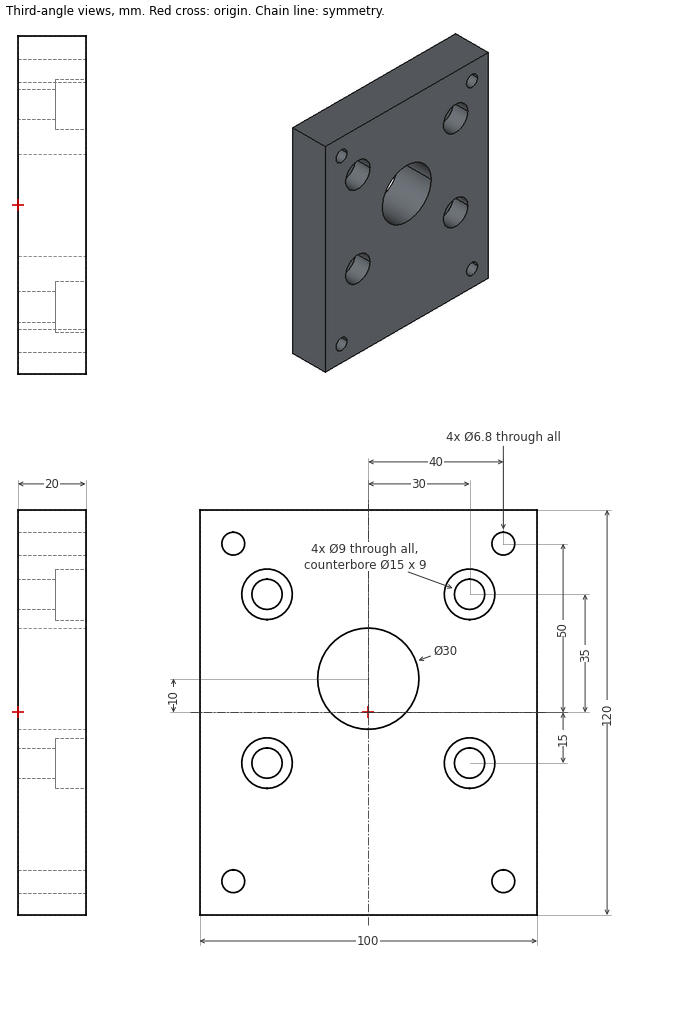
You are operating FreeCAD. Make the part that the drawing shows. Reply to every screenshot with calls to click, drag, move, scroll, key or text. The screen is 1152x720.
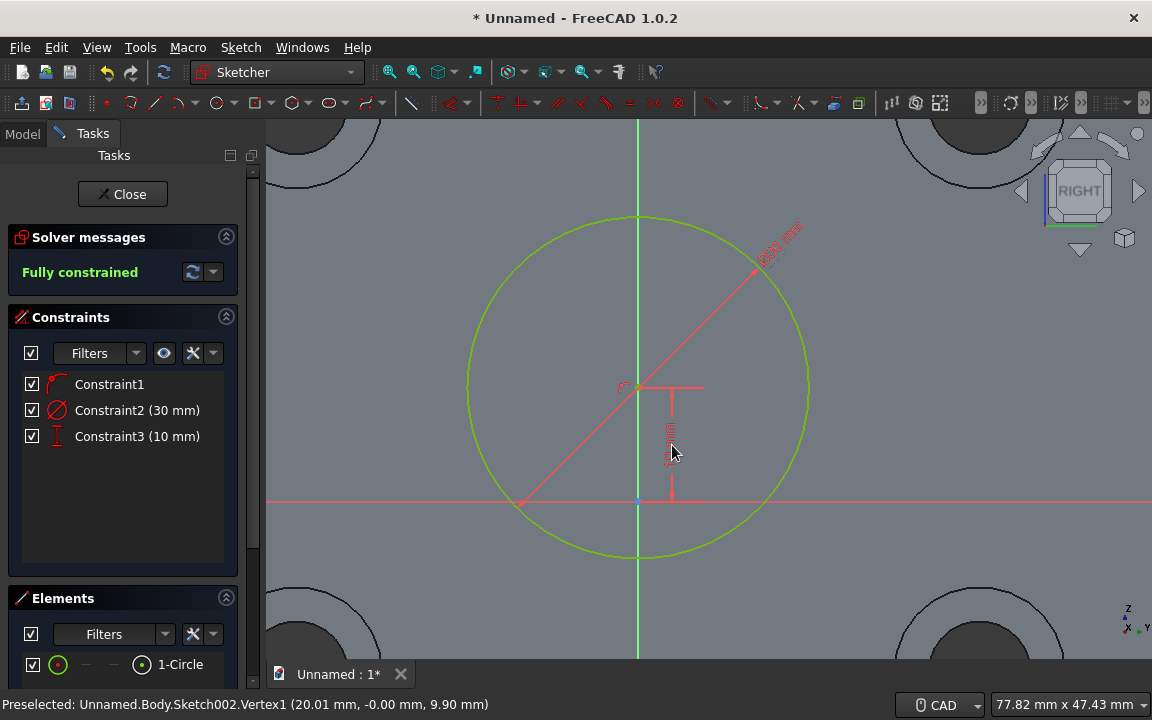
click(123, 194)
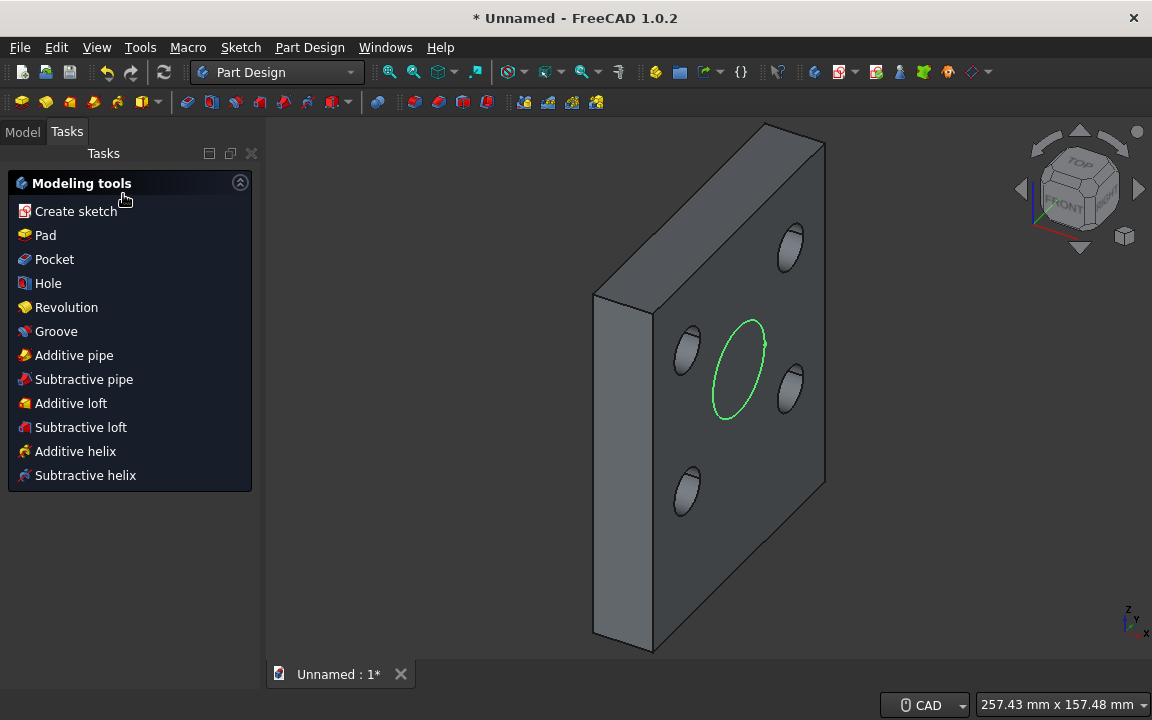
click(188, 102)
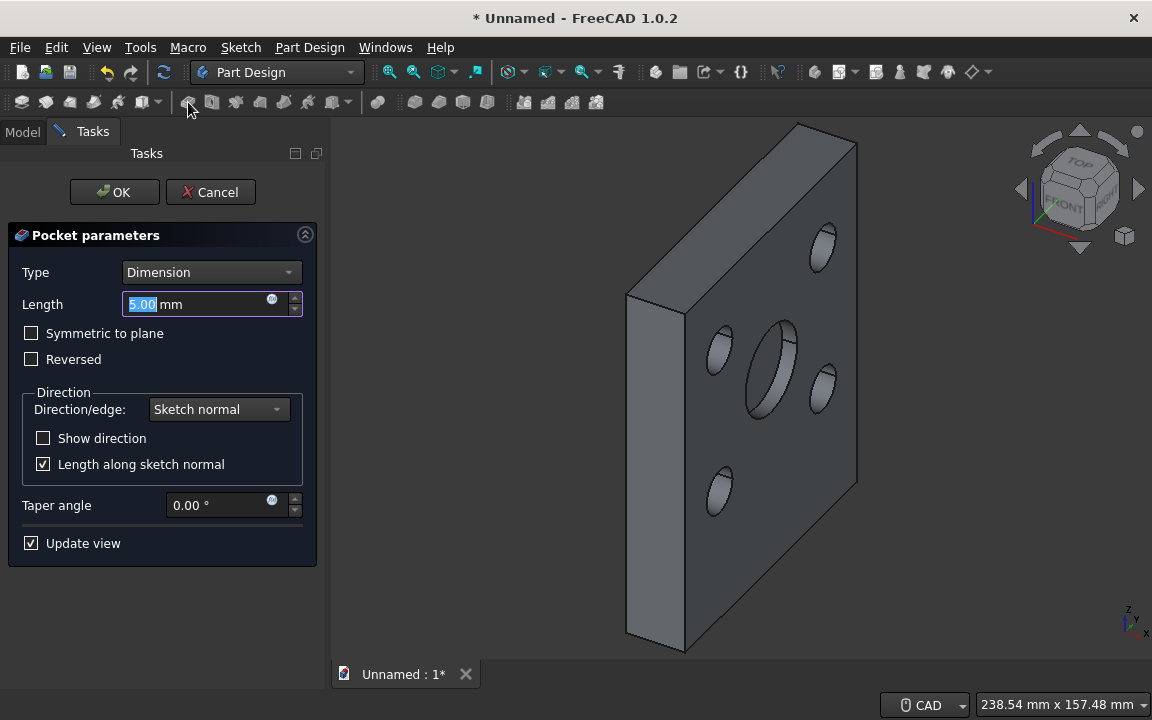
click(212, 272)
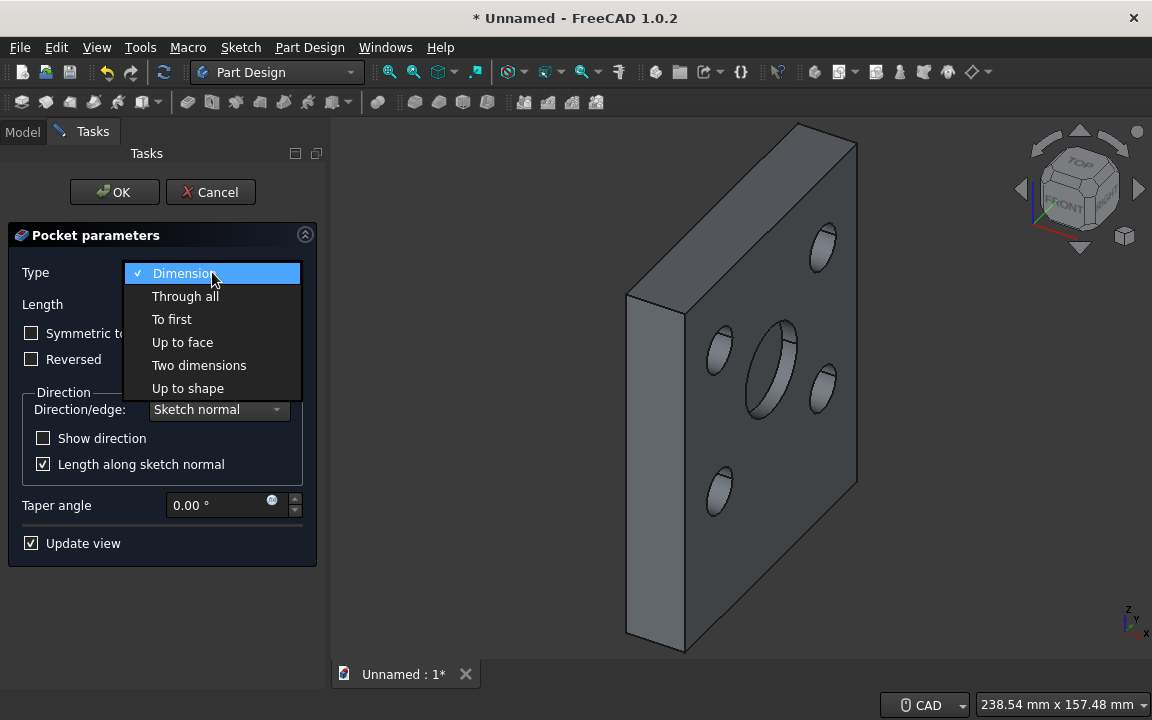
click(212, 296)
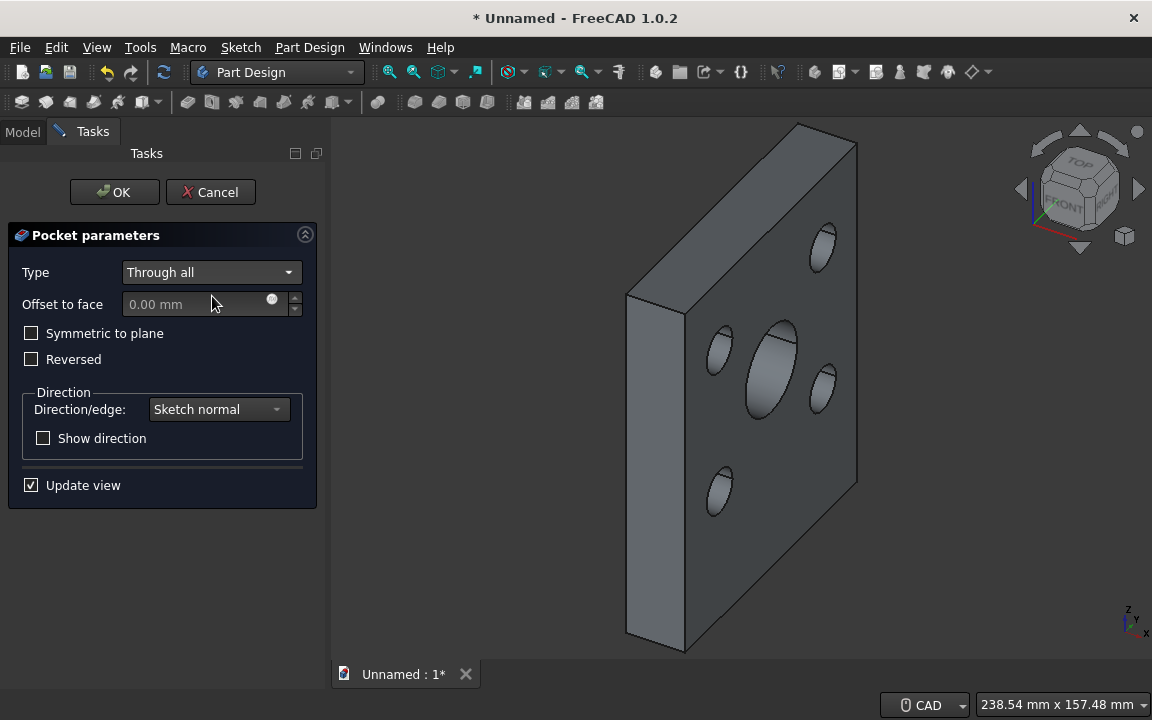
click(115, 192)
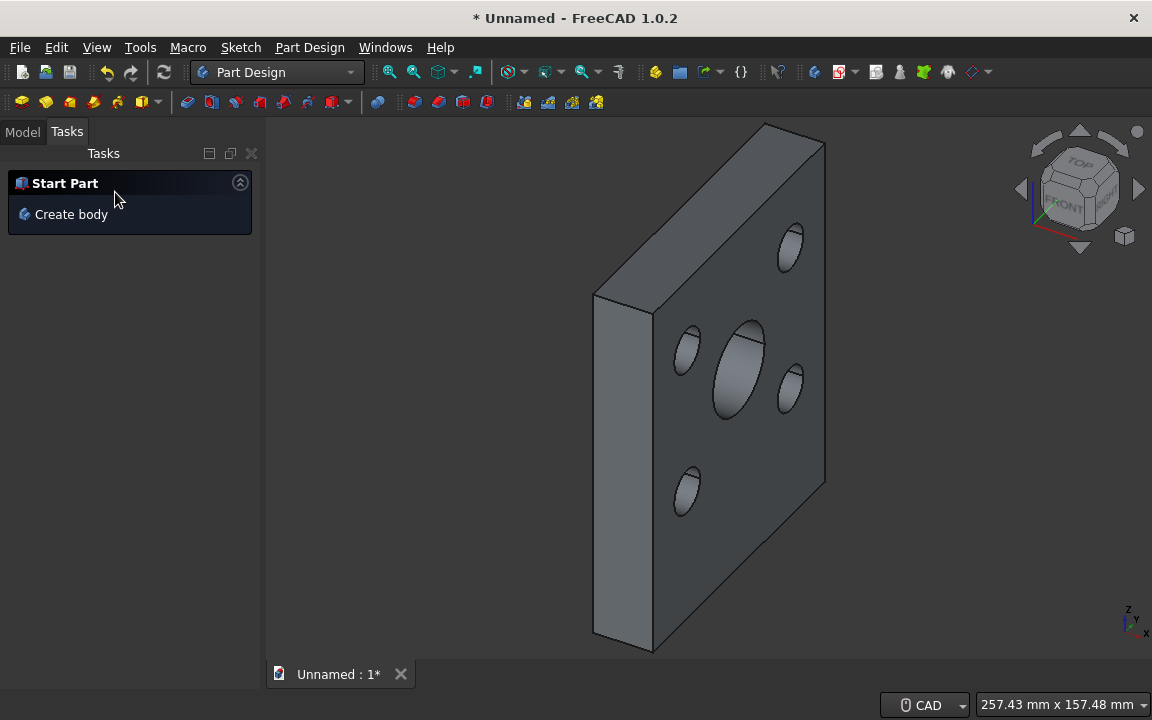
click(739, 494)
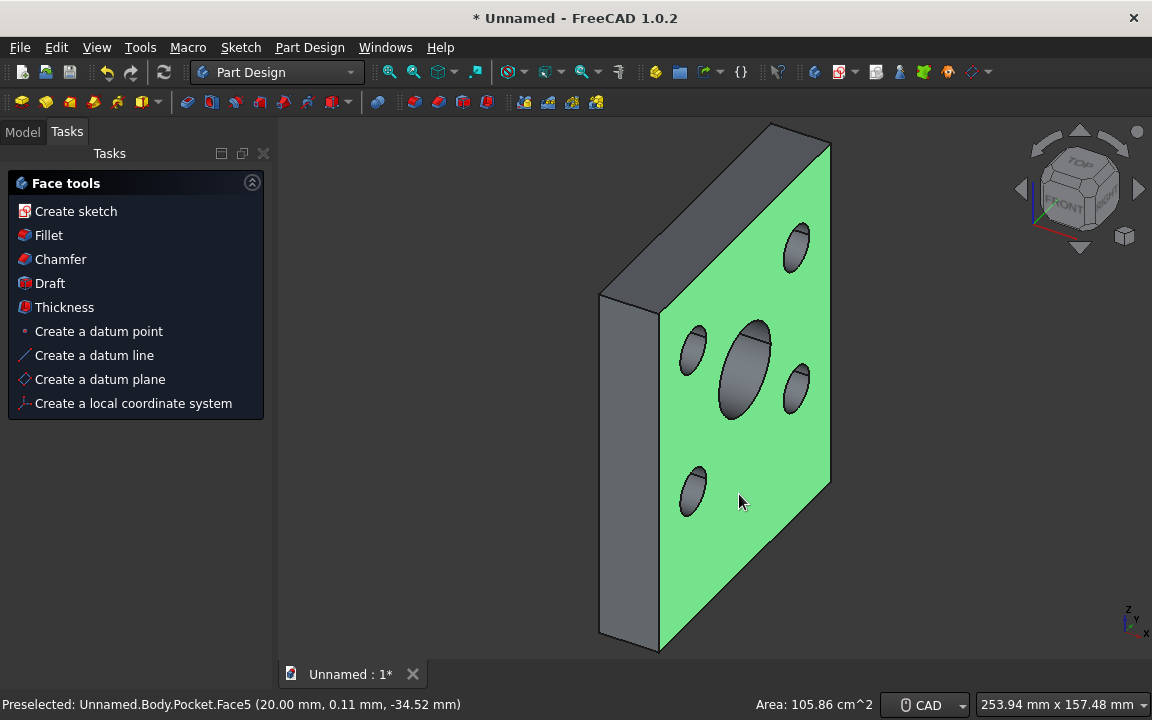
click(840, 72)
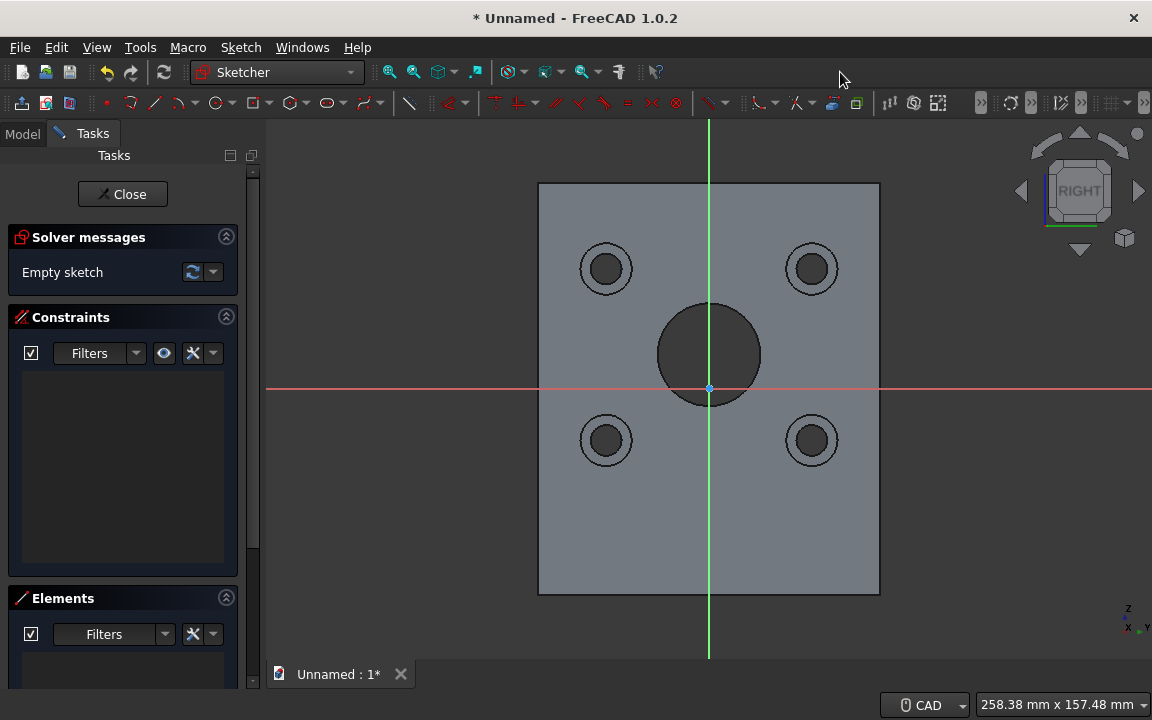
click(216, 104)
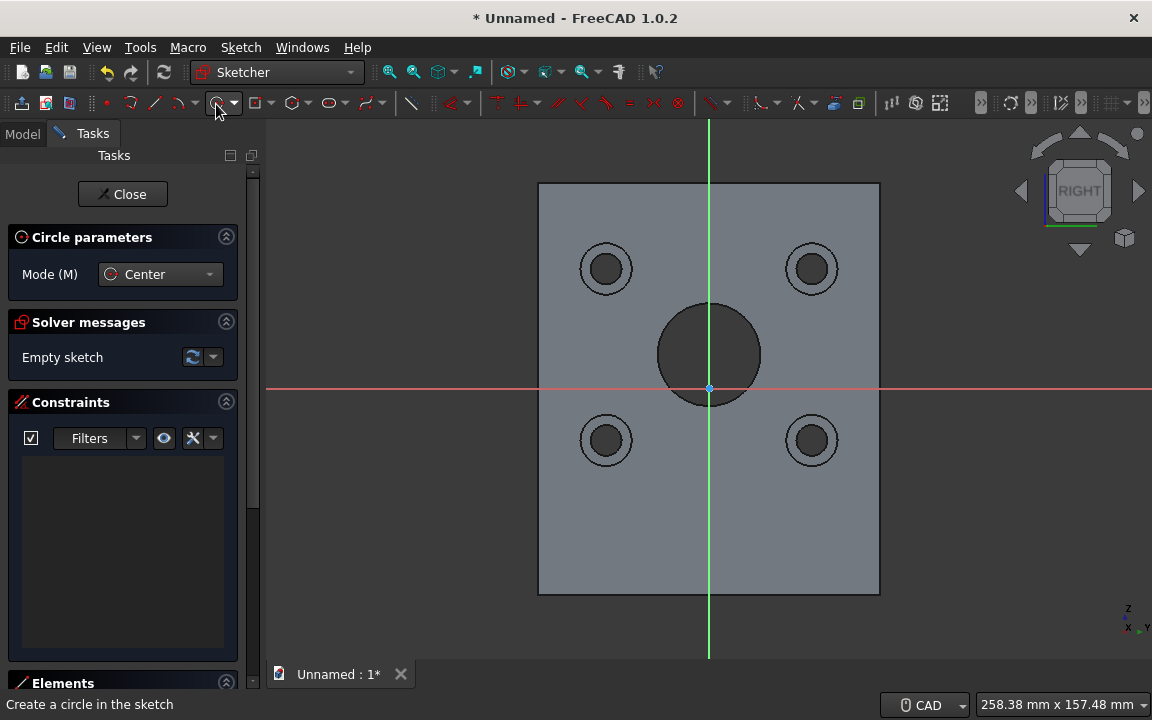
scroll(846, 218, up, 4)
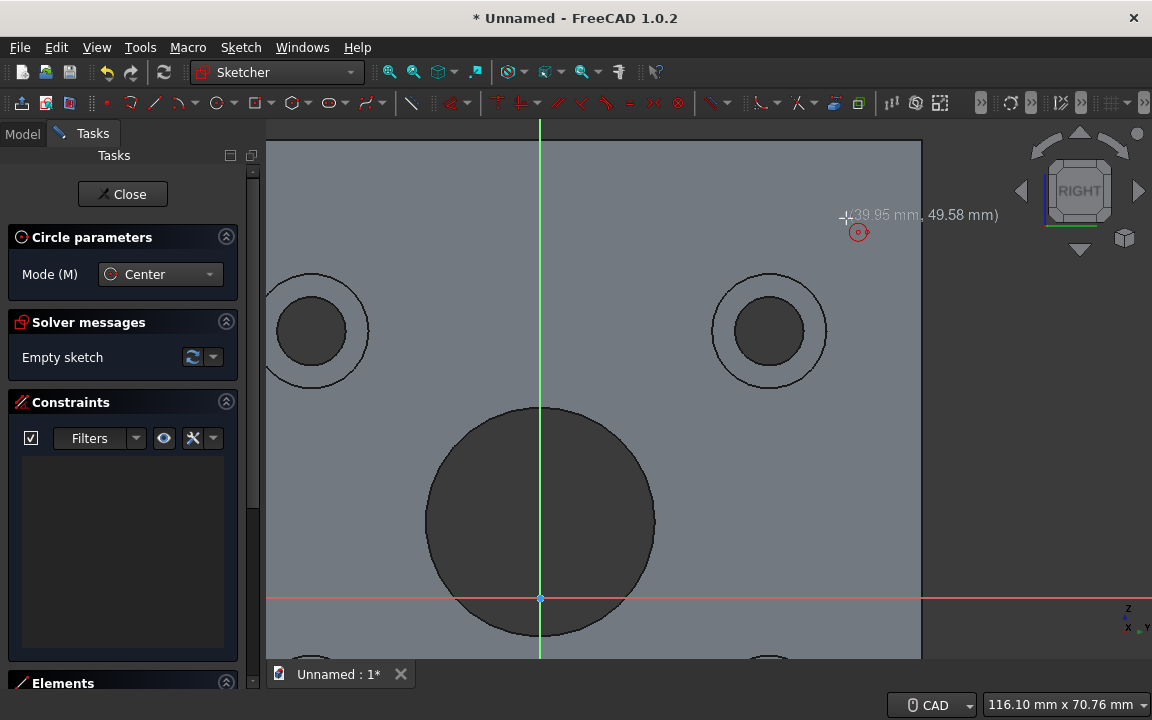
click(846, 217)
click(864, 198)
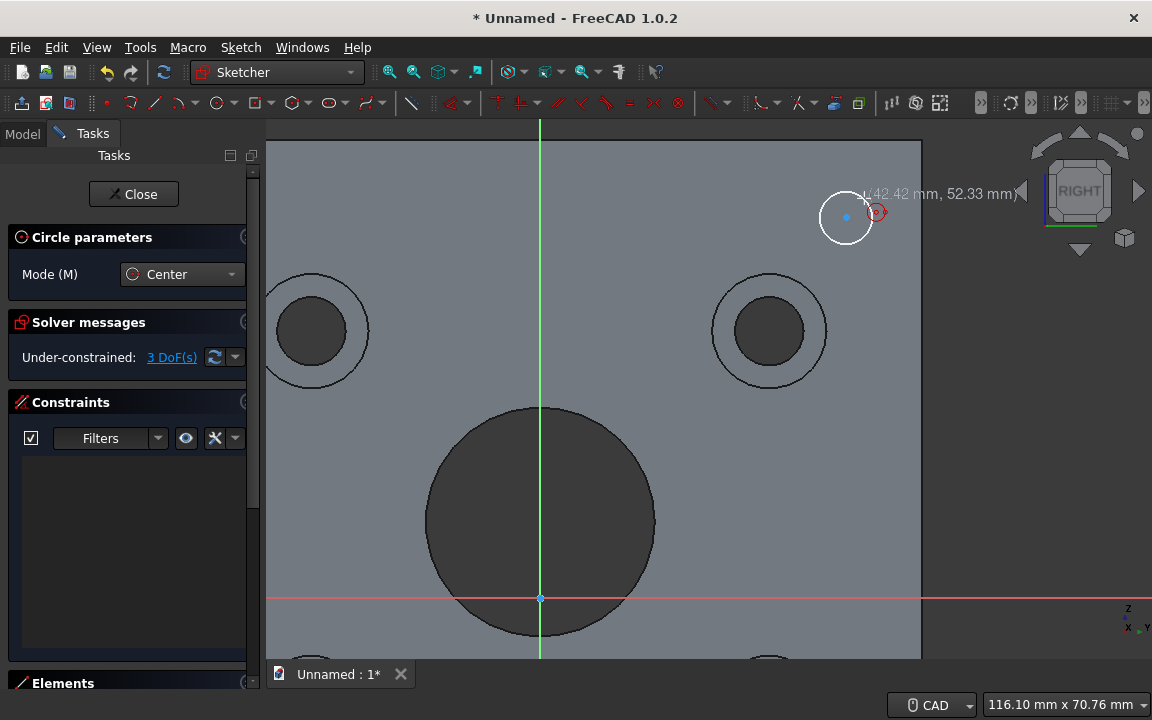
scroll(722, 218, down, 4)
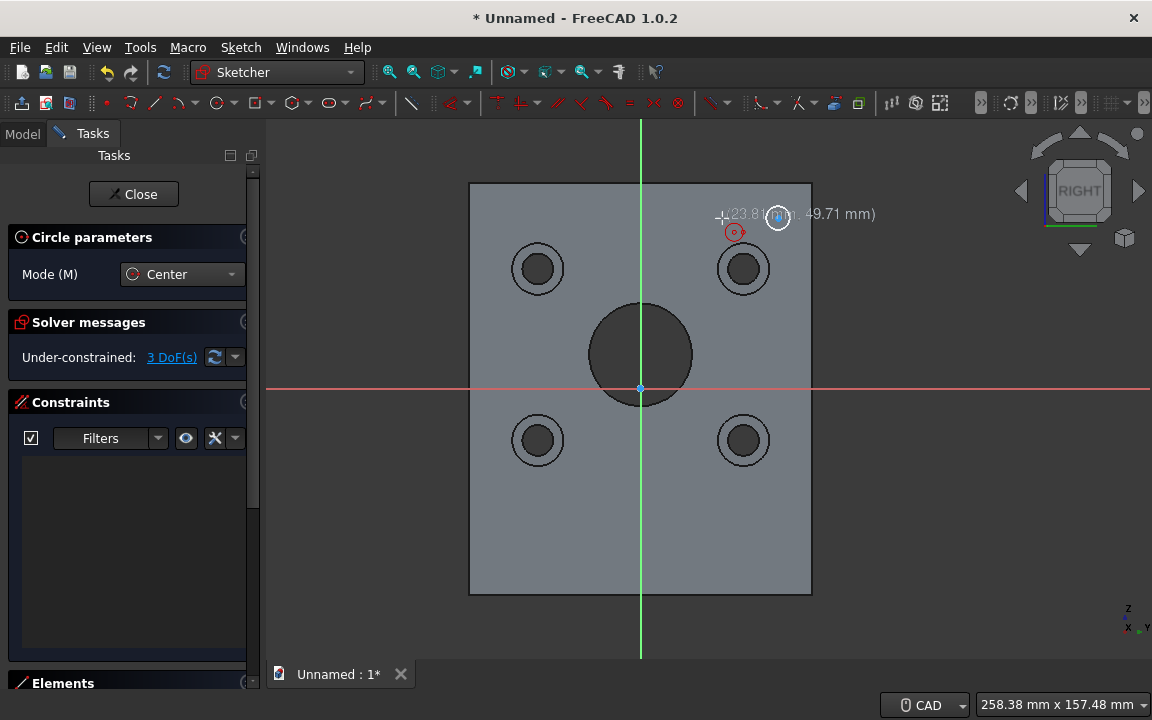
scroll(503, 218, up, 4)